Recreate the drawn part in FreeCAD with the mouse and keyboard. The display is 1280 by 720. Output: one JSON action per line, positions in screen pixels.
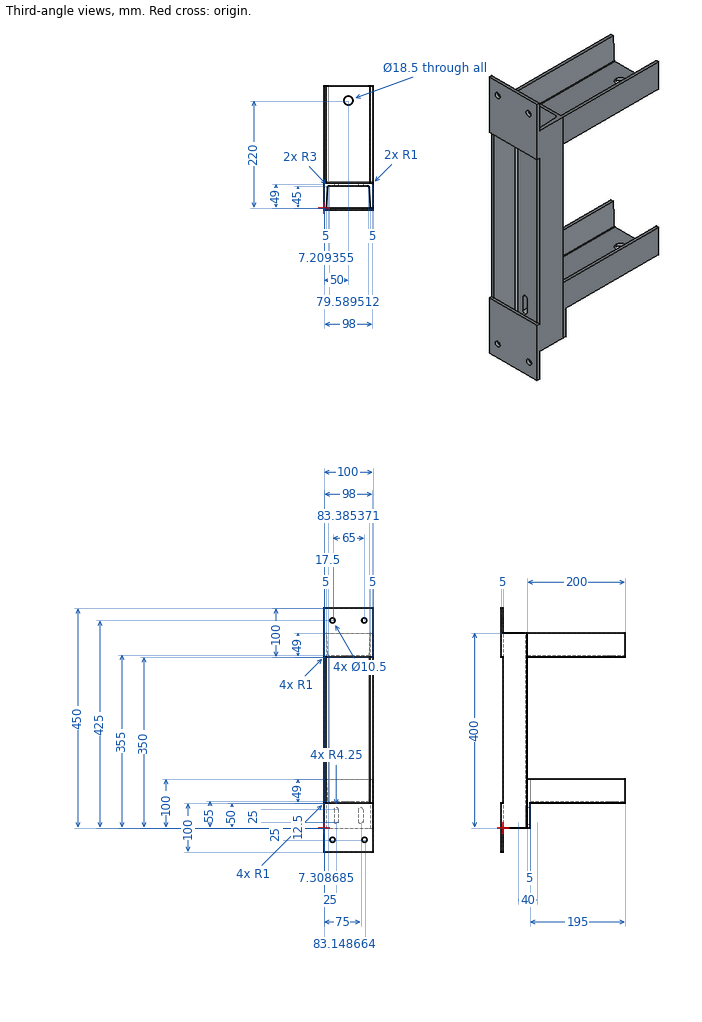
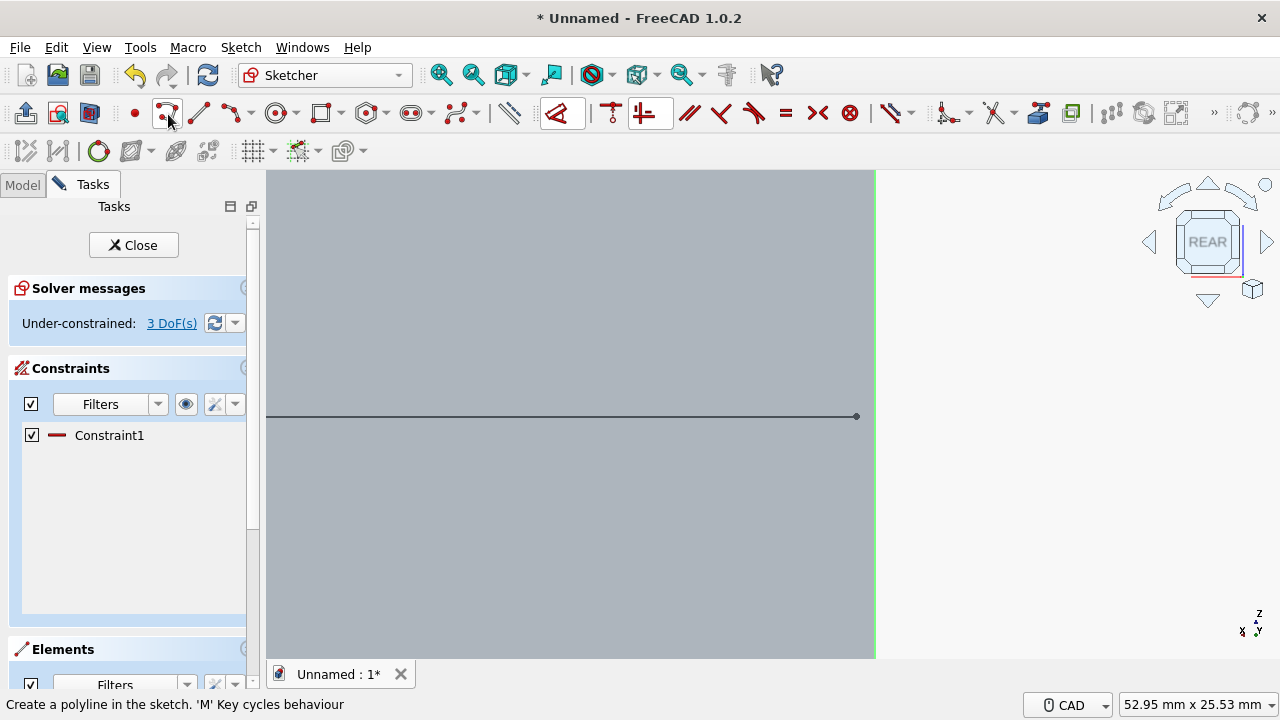
{"action": "left_click", "coordinate": [875, 390]}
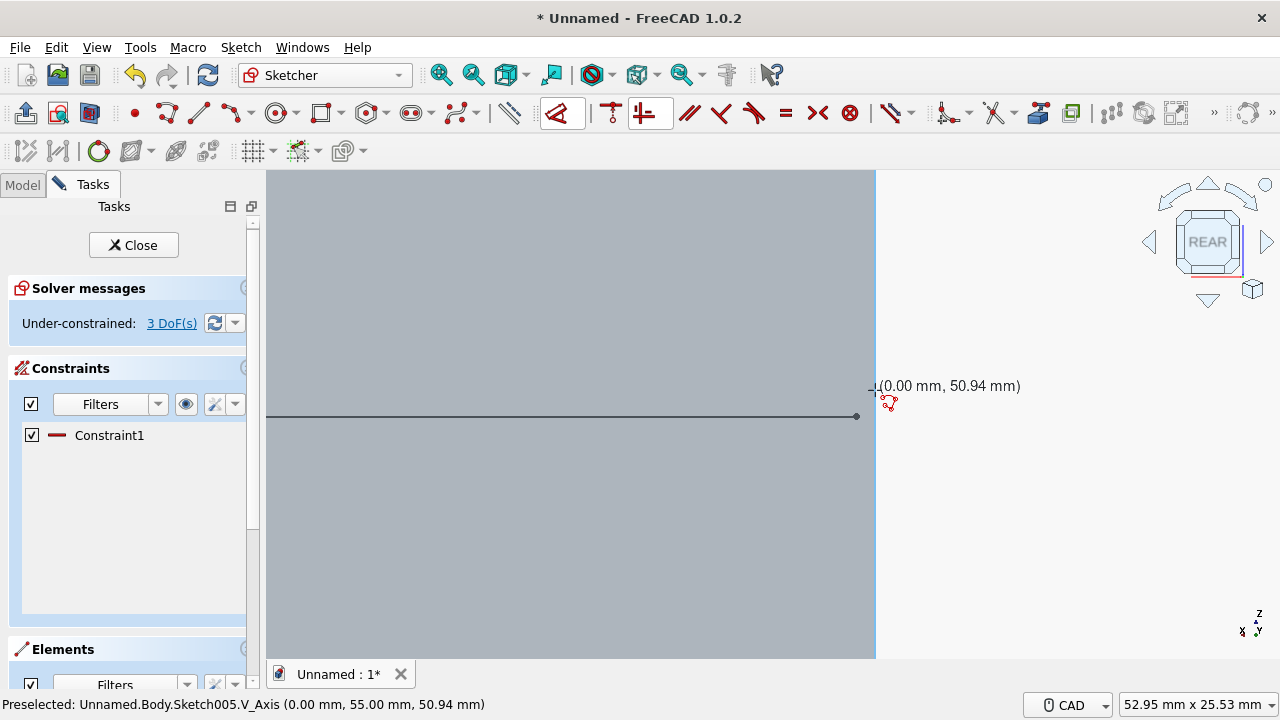
{"action": "scroll", "coordinate": [860, 416], "scroll_direction": "down", "scroll_amount": 9}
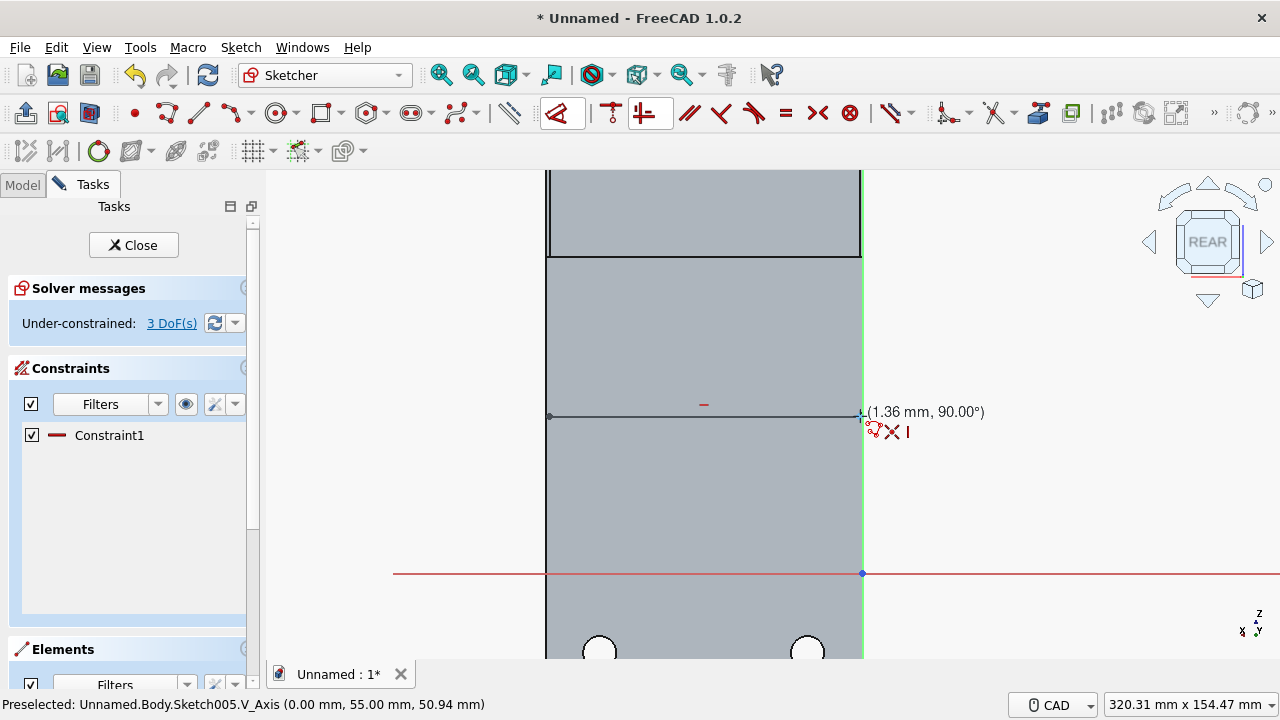
{"action": "left_click", "coordinate": [854, 257]}
{"action": "left_click", "coordinate": [847, 257]}
{"action": "left_click", "coordinate": [839, 396]}
{"action": "right_click", "coordinate": [839, 396]}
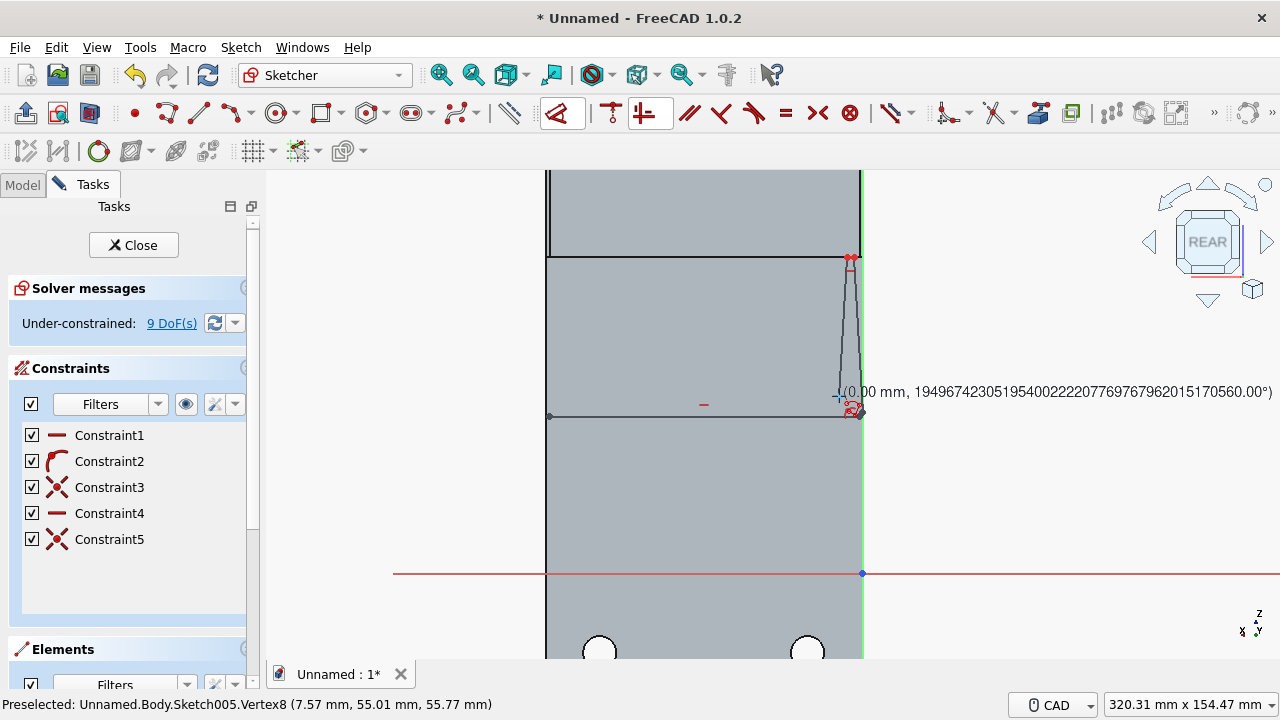
{"action": "key", "text": "g l"}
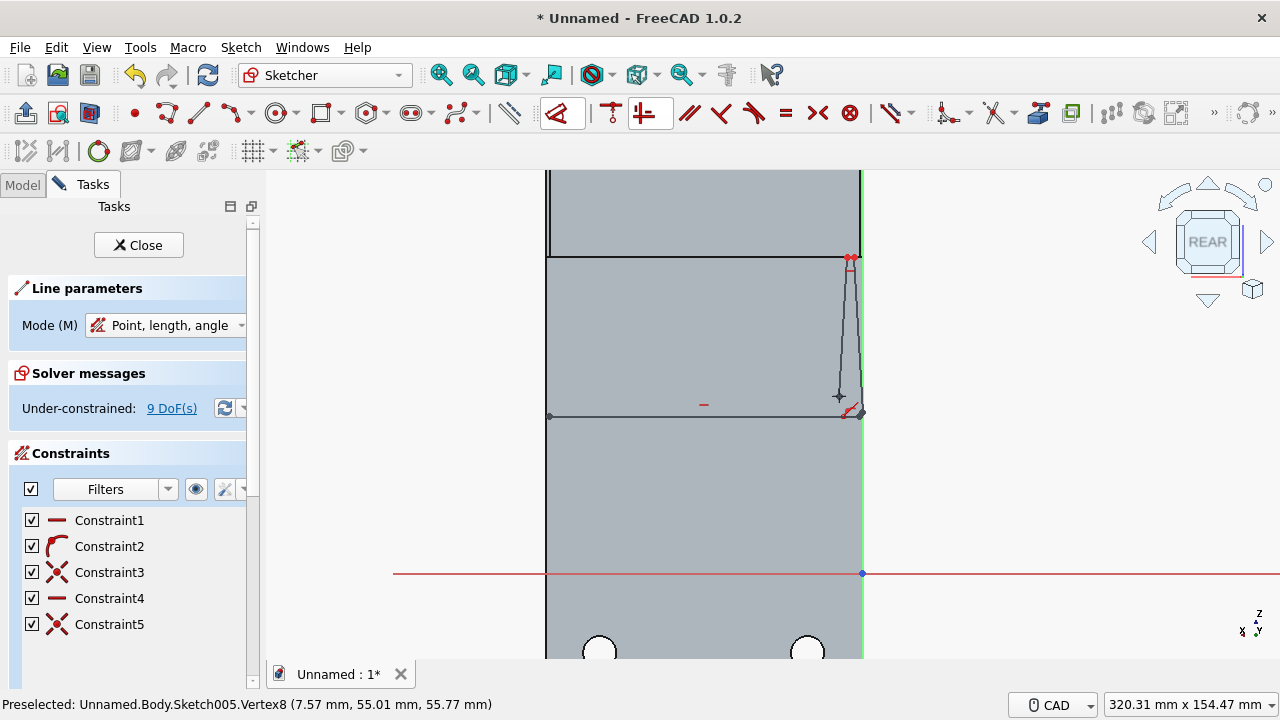
{"action": "scroll", "coordinate": [837, 399], "scroll_direction": "up", "scroll_amount": 7}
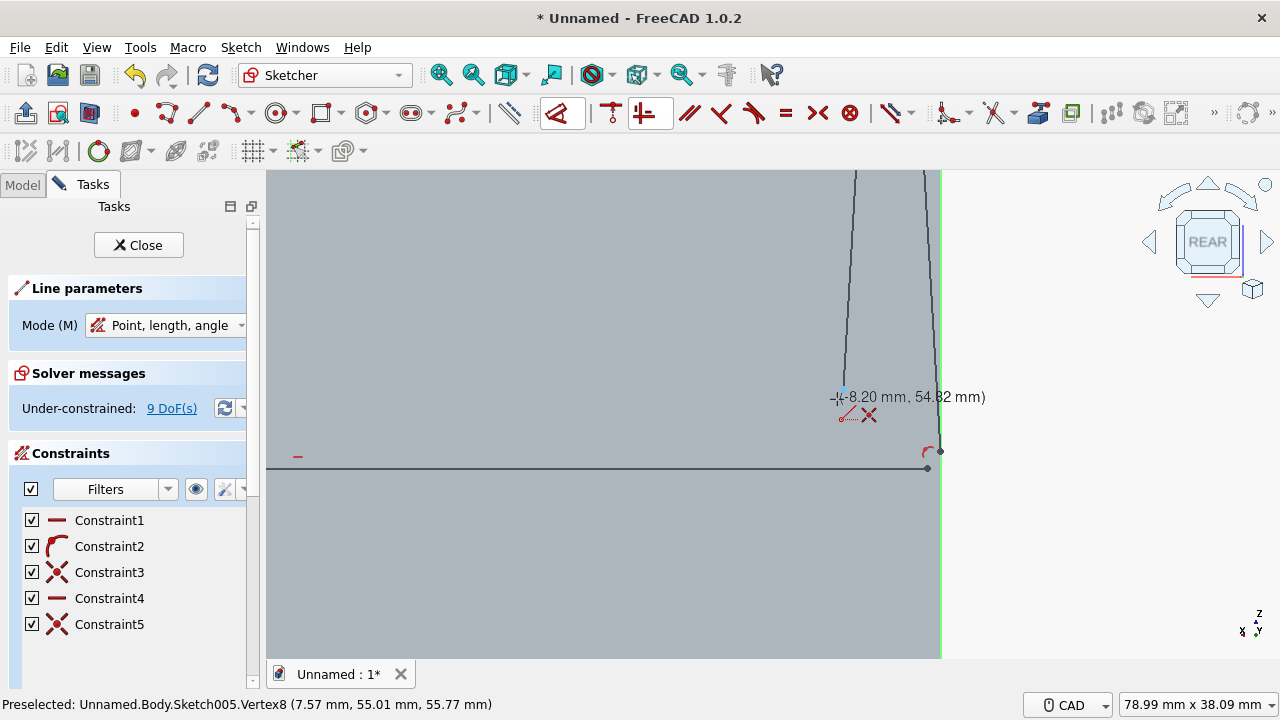
{"action": "left_click", "coordinate": [834, 399]}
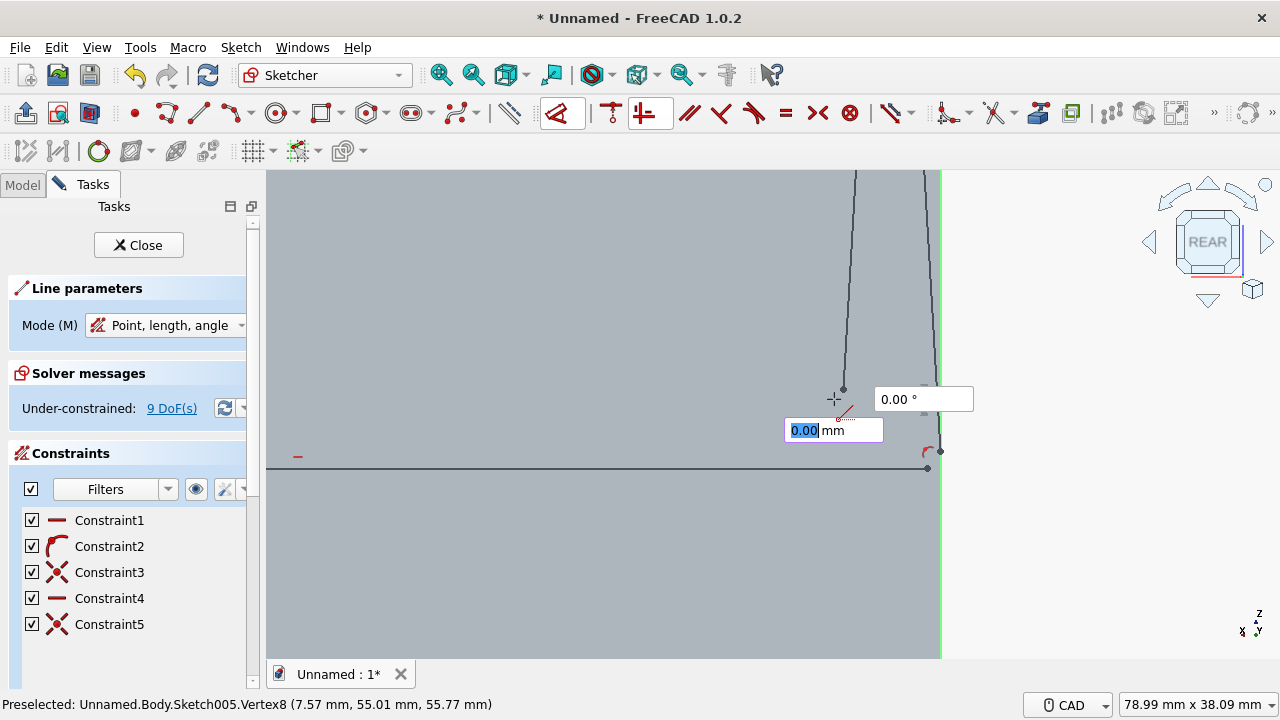
{"action": "scroll", "coordinate": [837, 398], "scroll_direction": "down", "scroll_amount": 7}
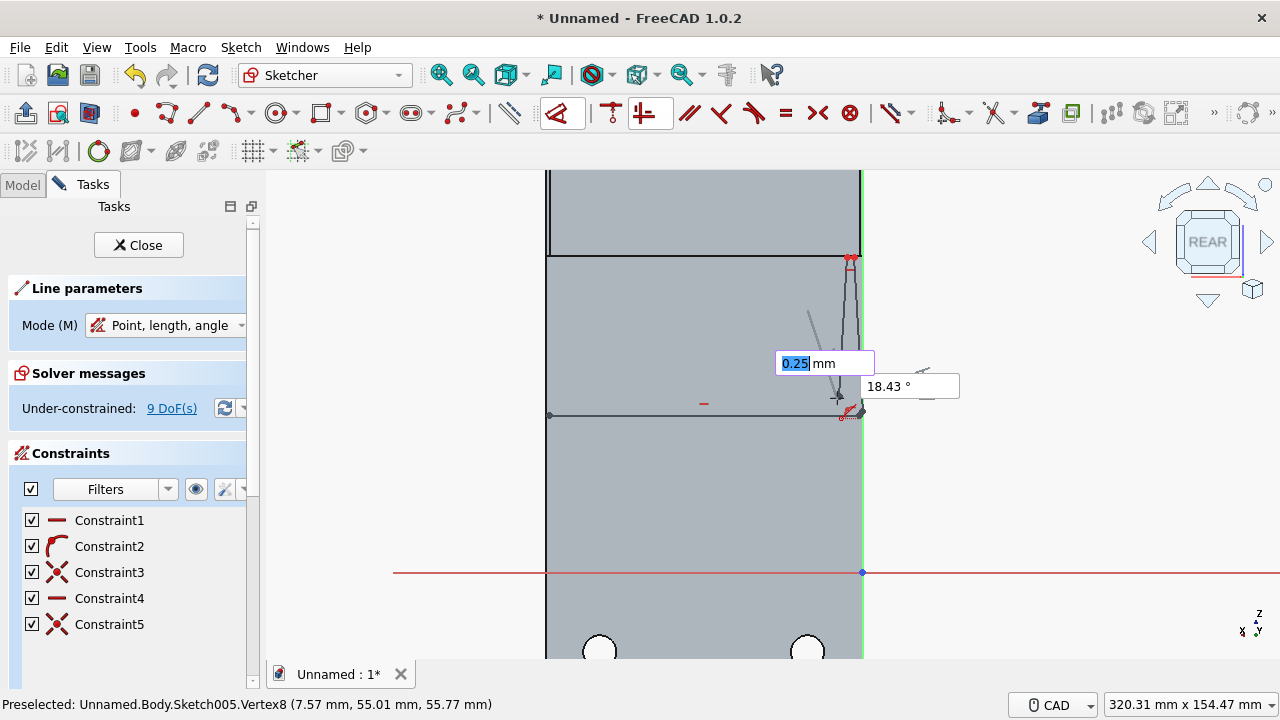
{"action": "left_click", "coordinate": [573, 399]}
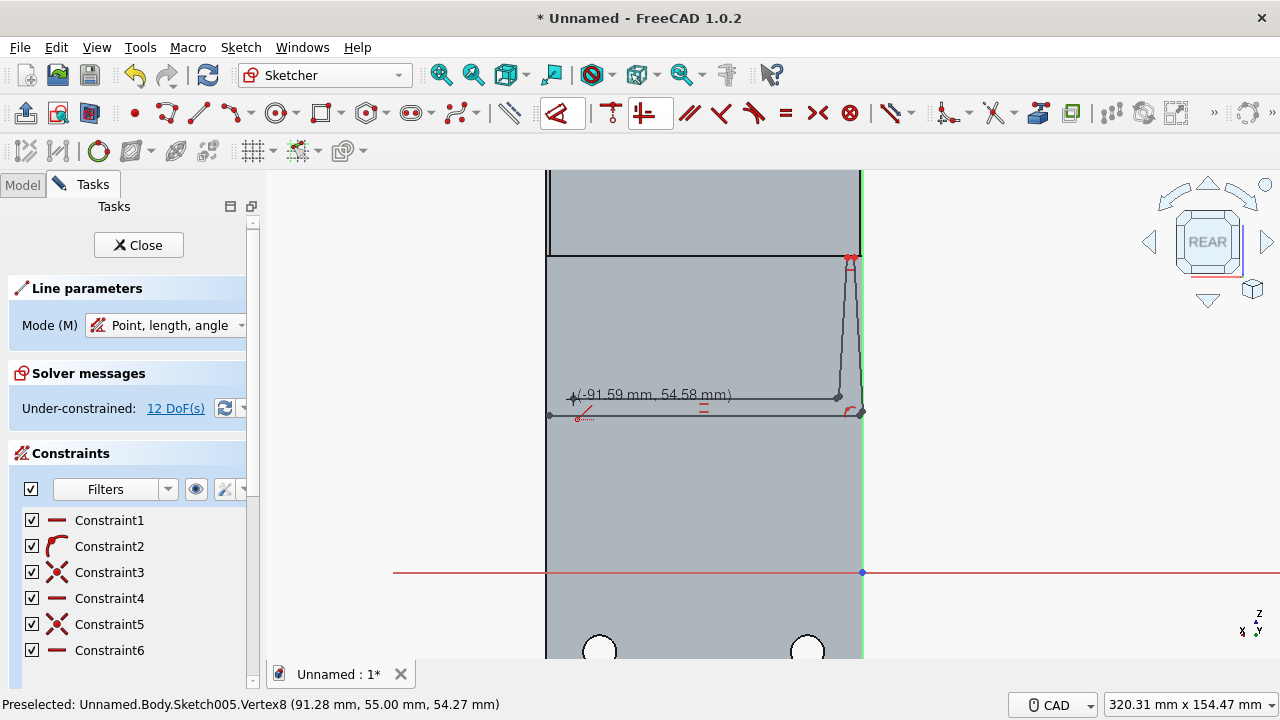
{"action": "left_click", "coordinate": [168, 114]}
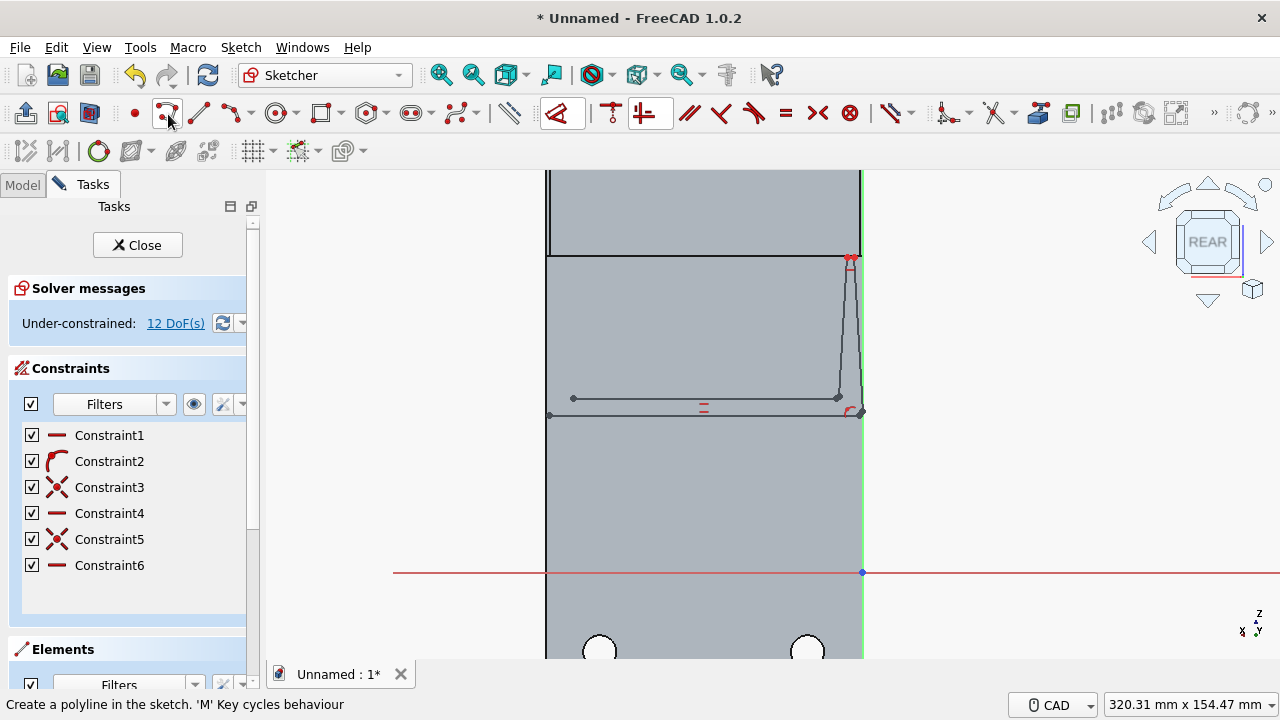
{"action": "scroll", "coordinate": [570, 396], "scroll_direction": "up", "scroll_amount": 7}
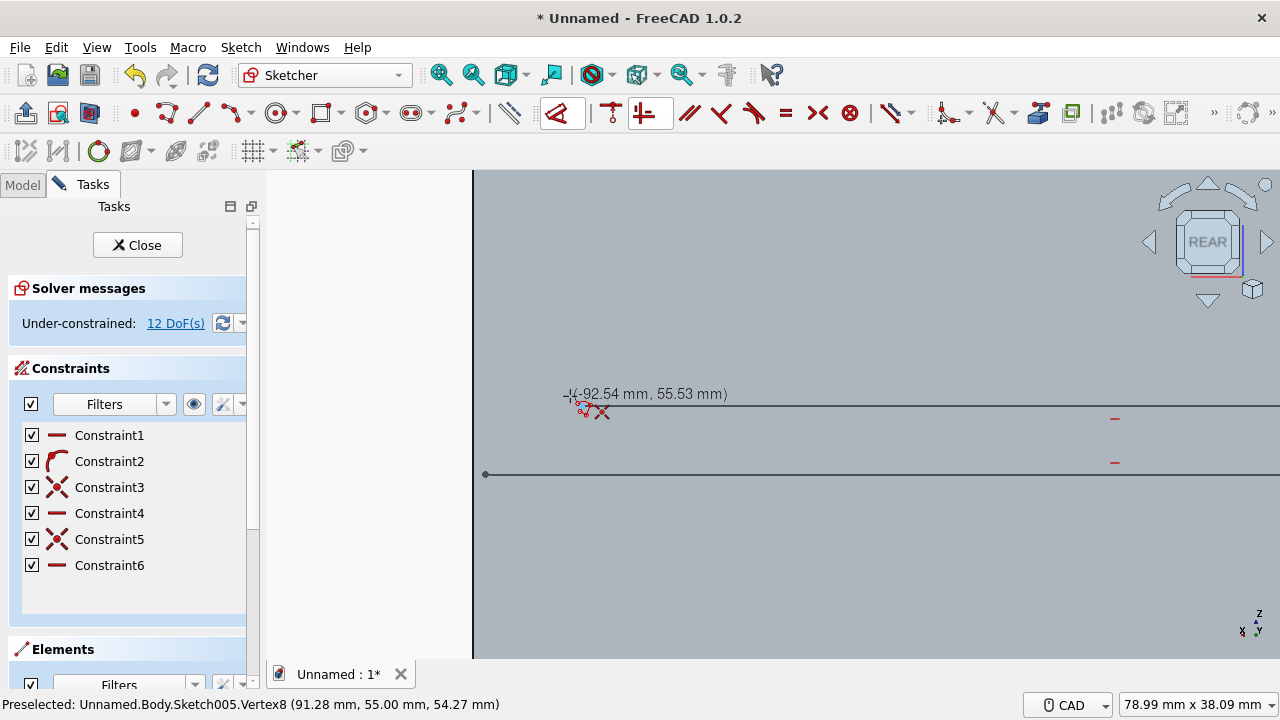
{"action": "left_click", "coordinate": [567, 393]}